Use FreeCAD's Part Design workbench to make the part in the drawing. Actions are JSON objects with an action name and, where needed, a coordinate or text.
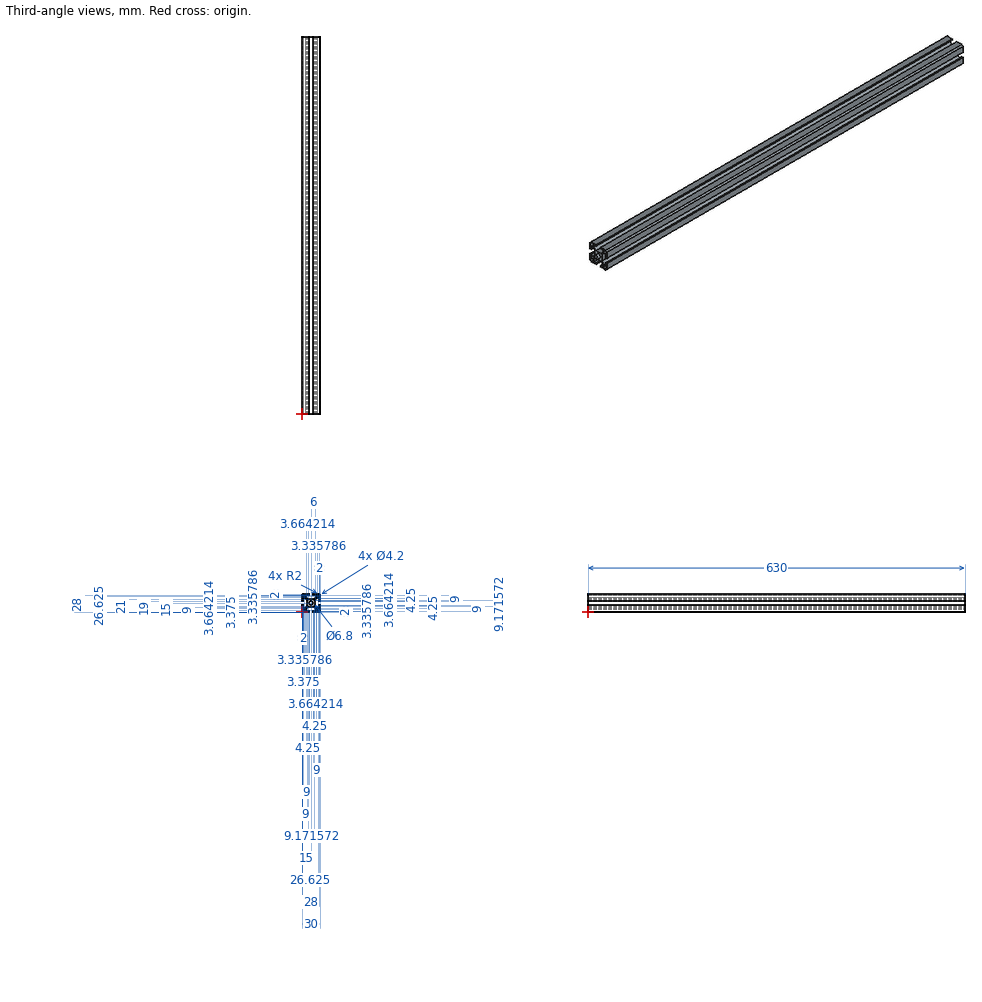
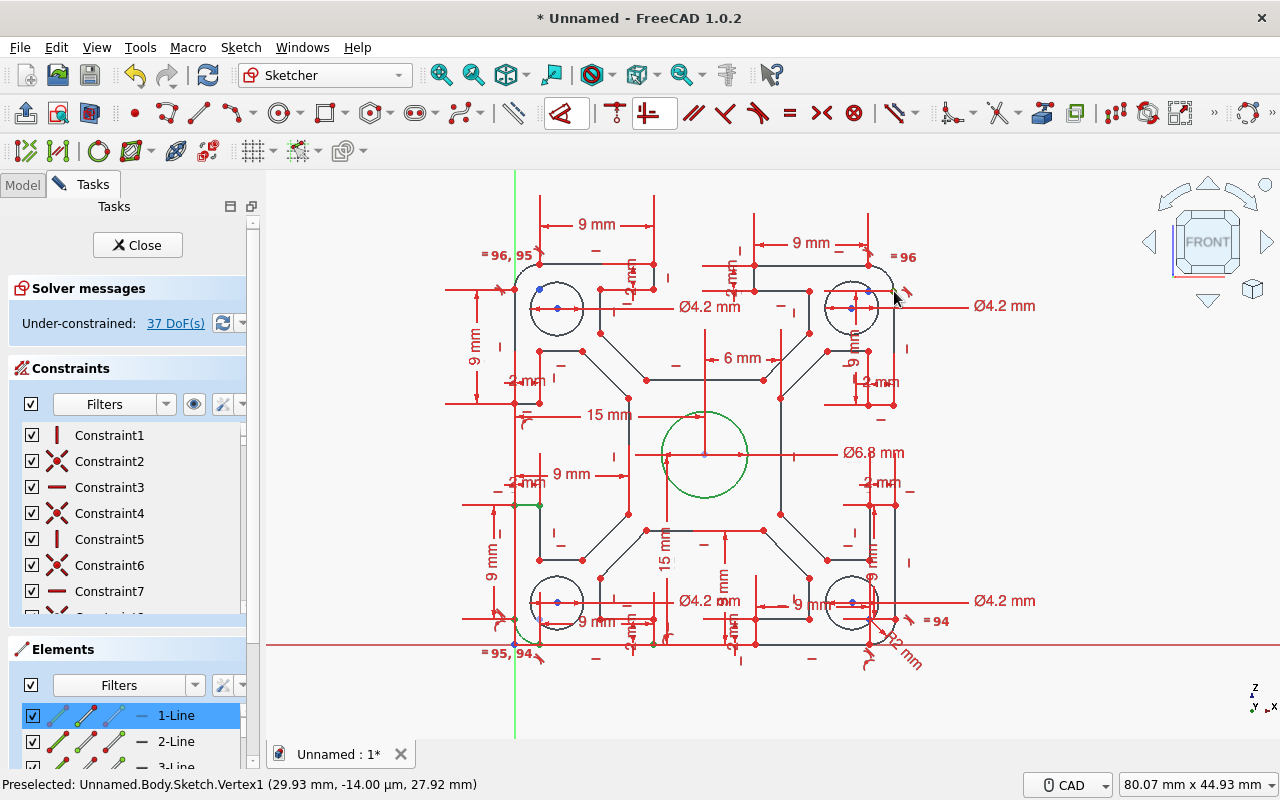
{"action": "left_click", "coordinate": [584, 114]}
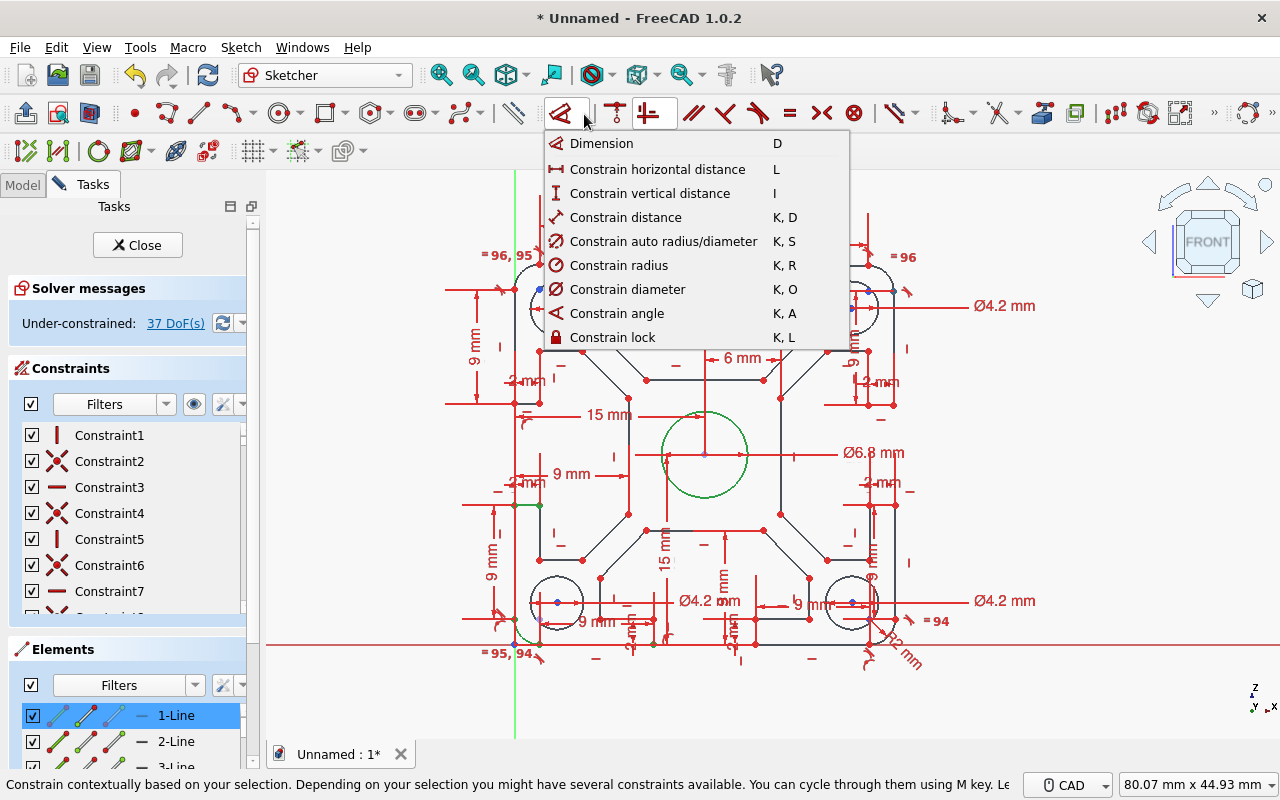
{"action": "left_click", "coordinate": [697, 169]}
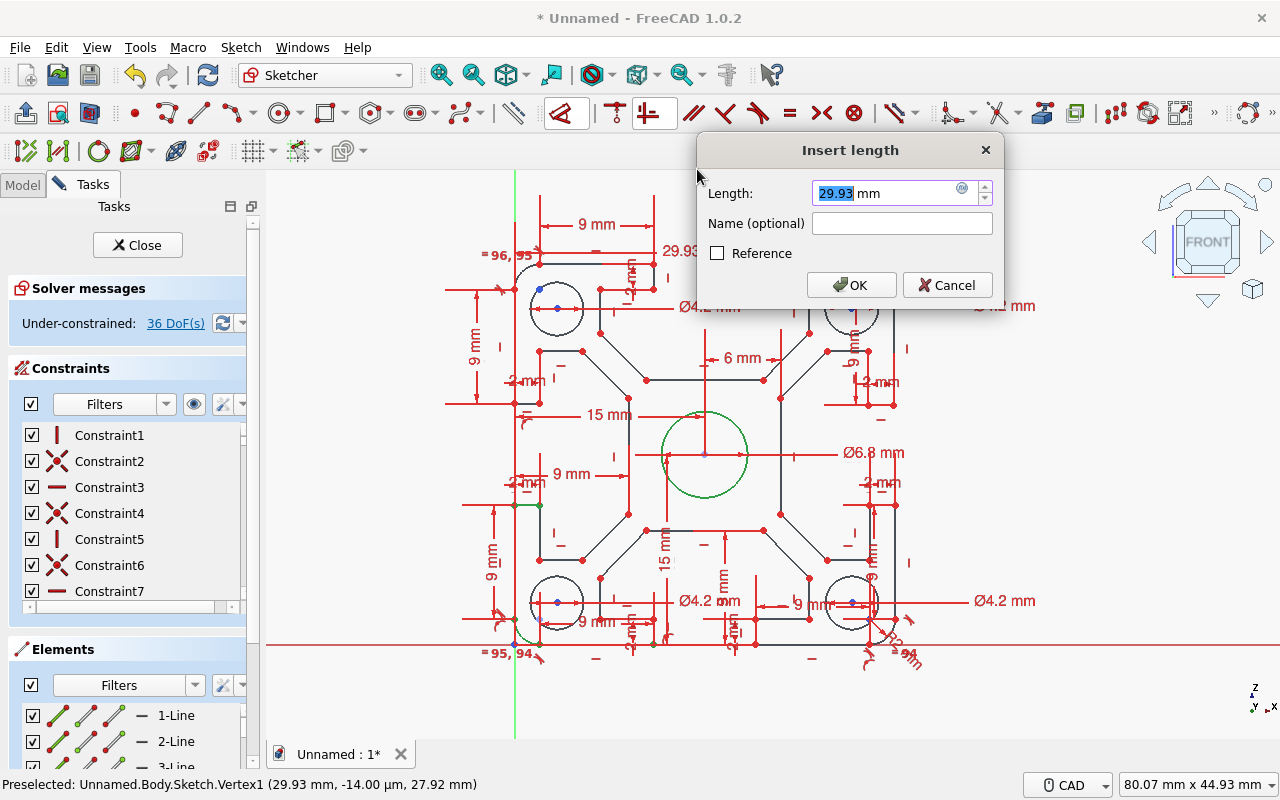
{"action": "type", "text": "30"}
{"action": "key", "text": "Return"}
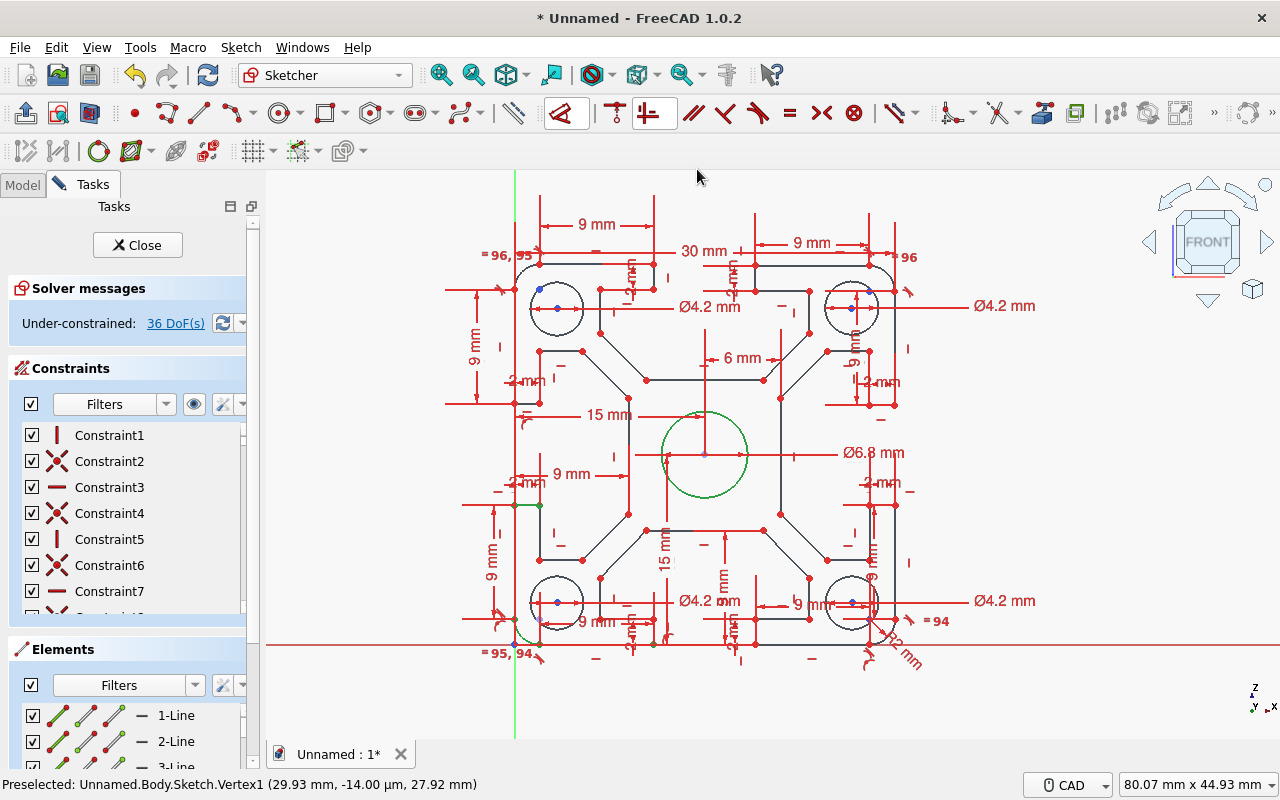
{"action": "left_click", "coordinate": [895, 291]}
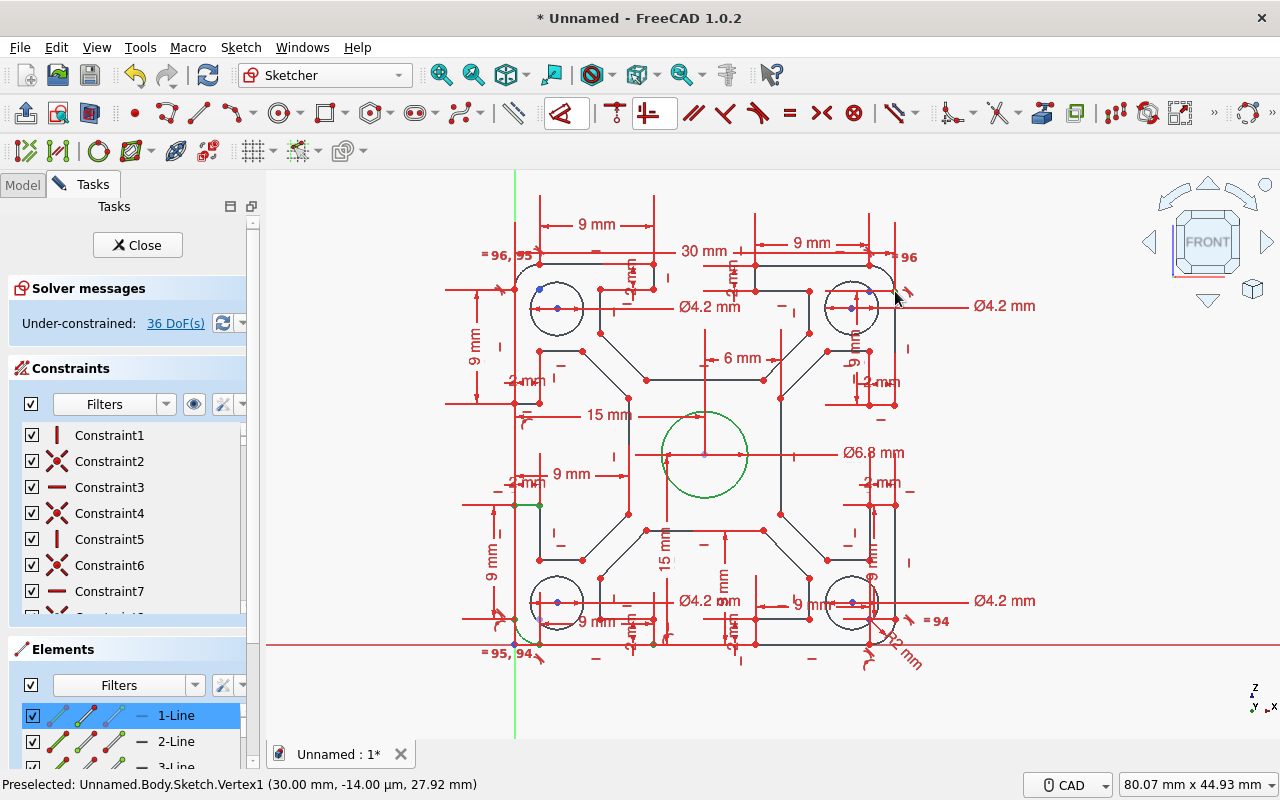
{"action": "key", "text": "i"}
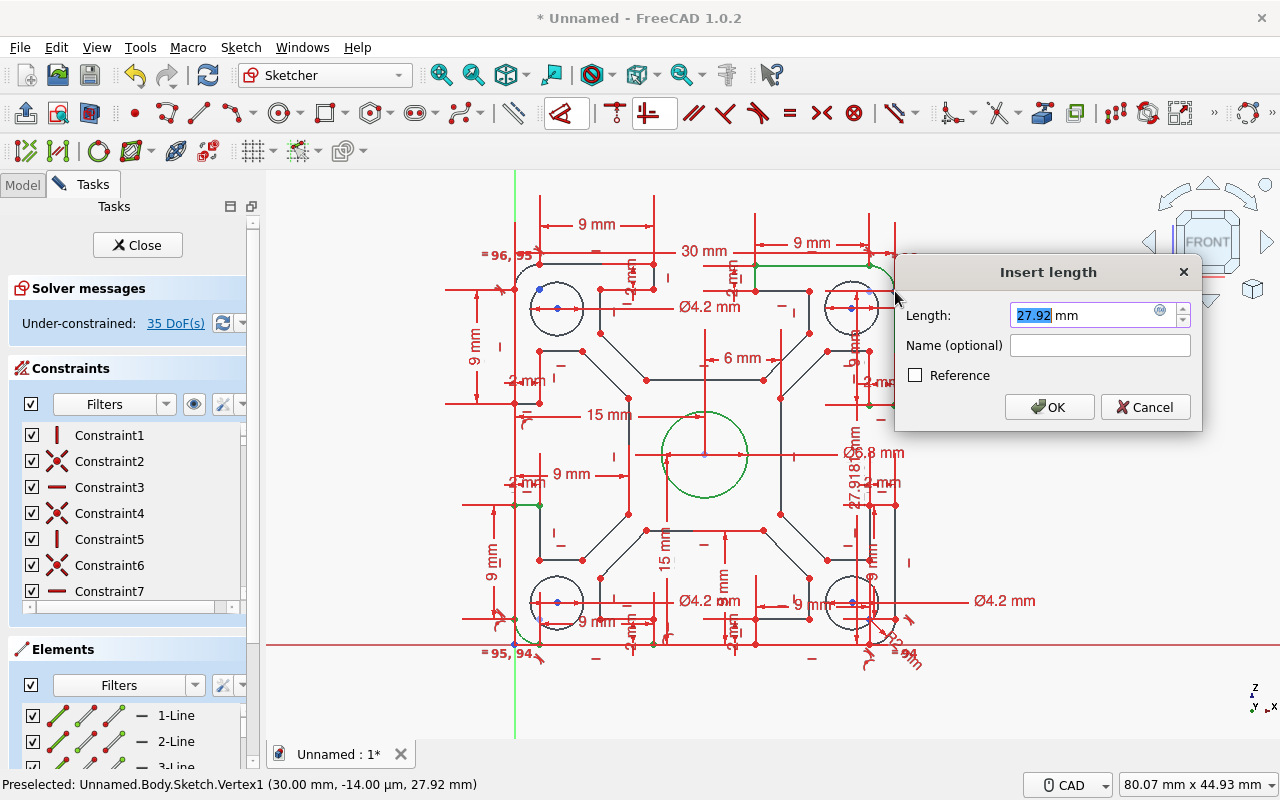
{"action": "type", "text": "28"}
{"action": "key", "text": "Return"}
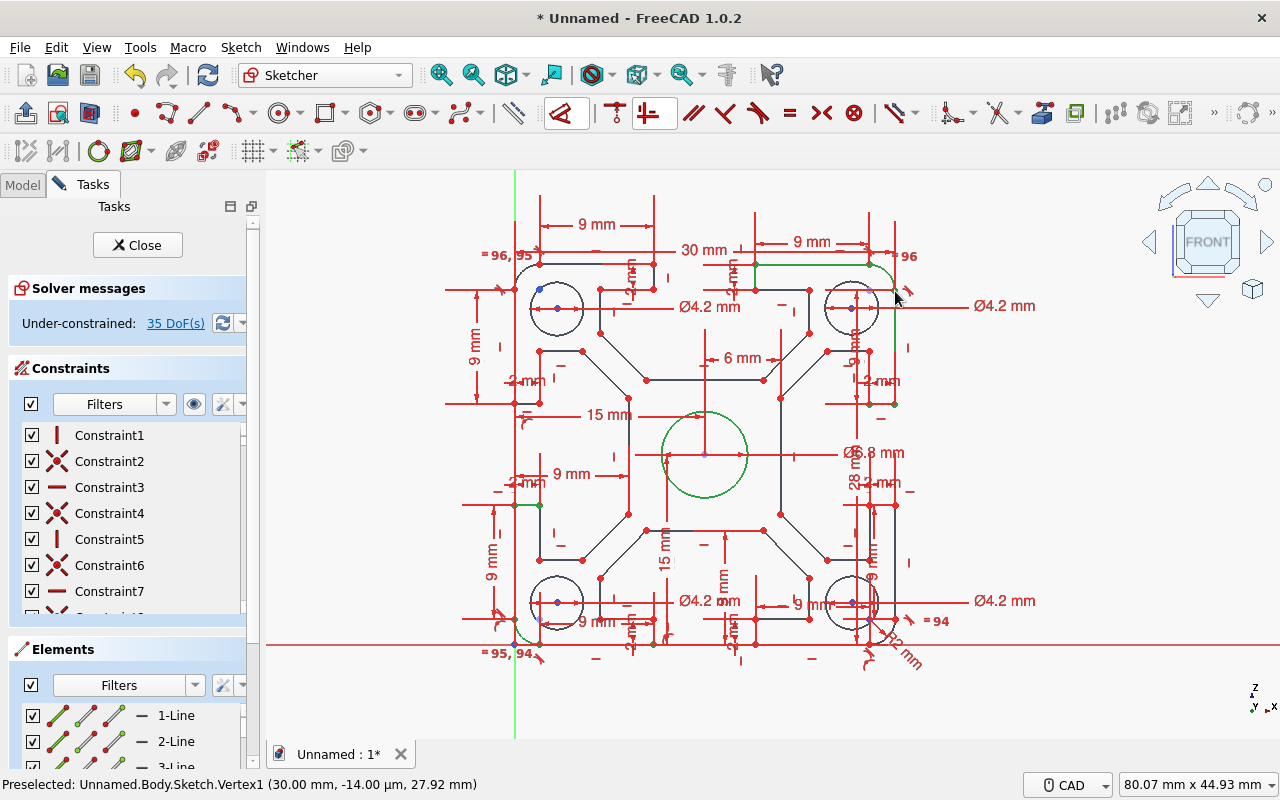
{"action": "left_click", "coordinate": [870, 560]}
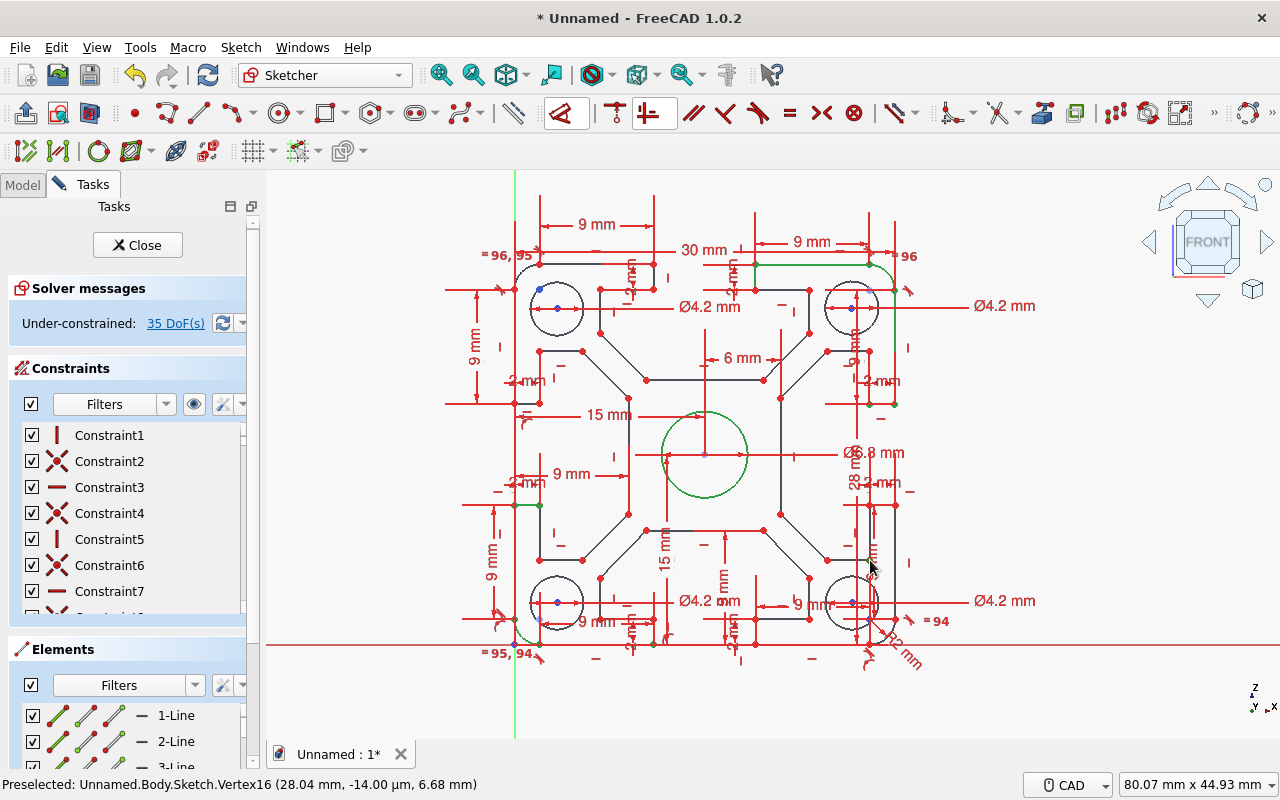
{"action": "key", "text": "l"}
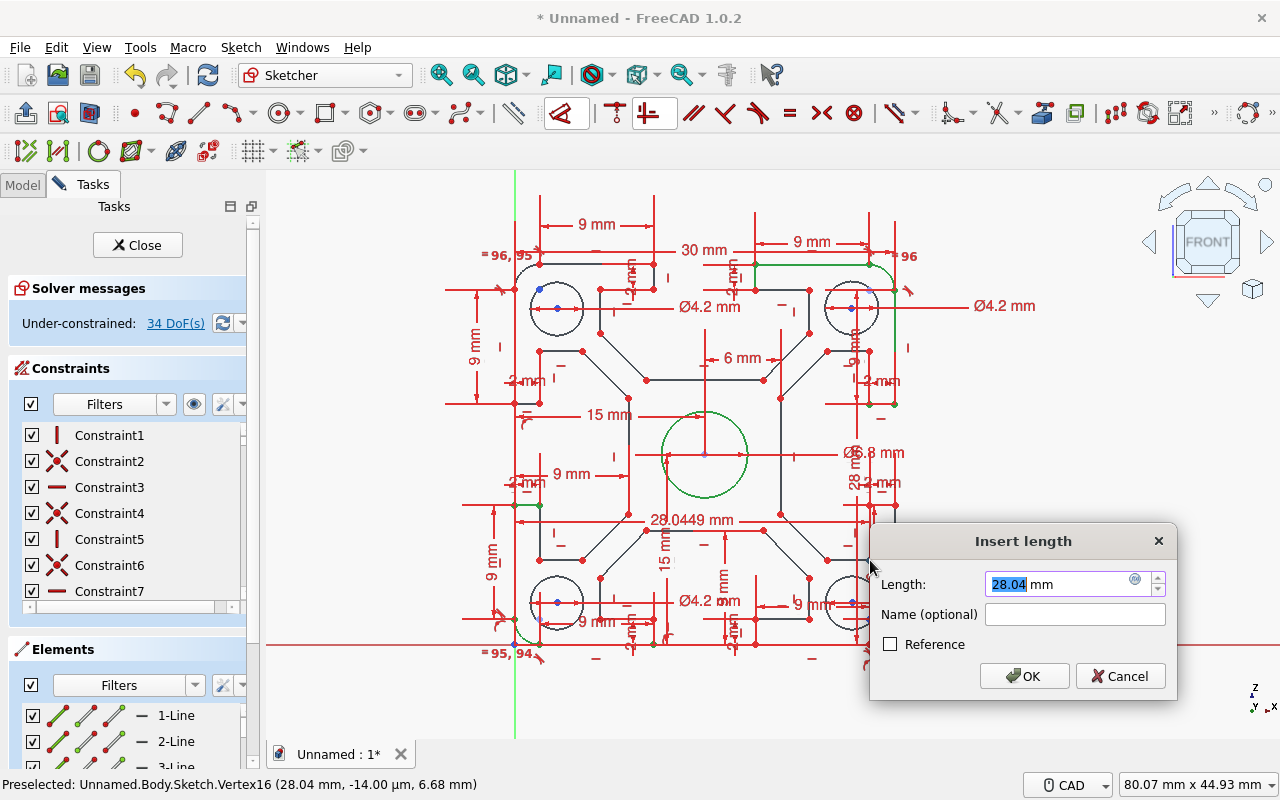
{"action": "type", "text": "28"}
{"action": "key", "text": "Return"}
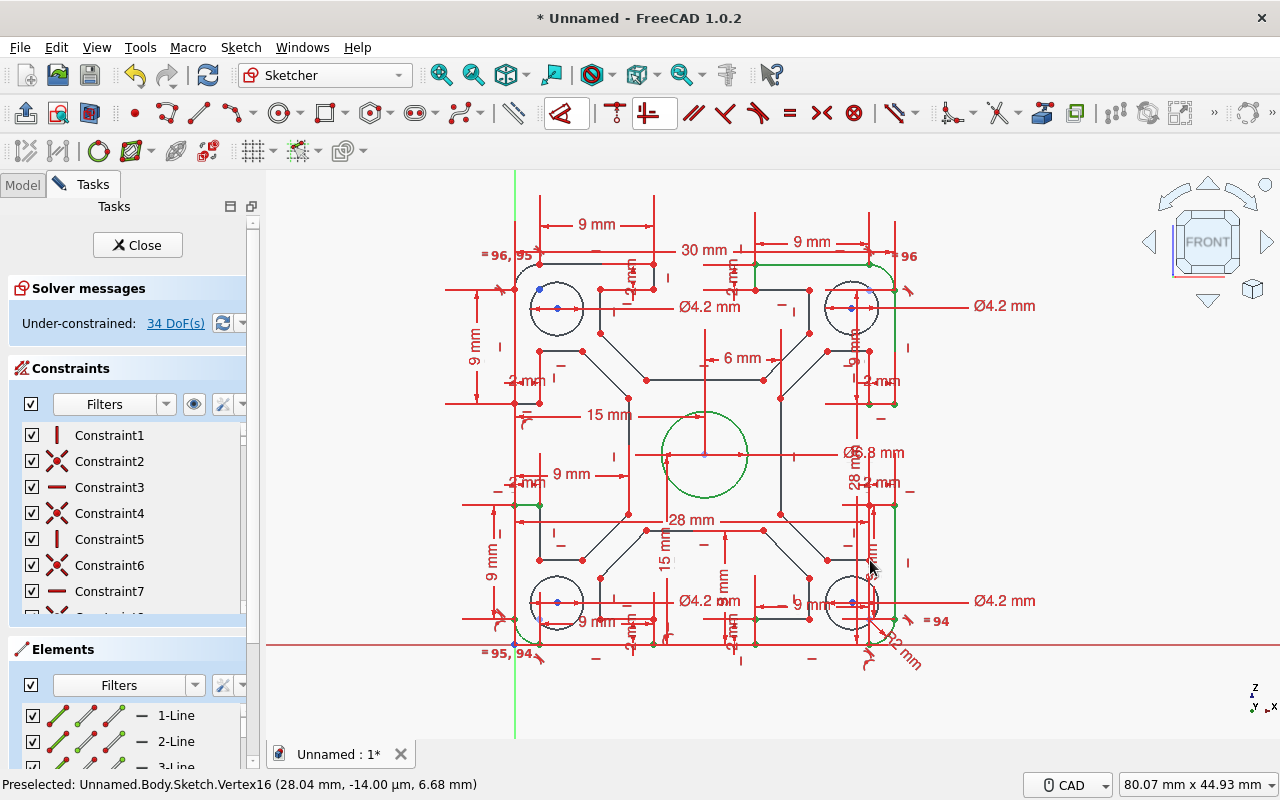
{"action": "left_click", "coordinate": [540, 404]}